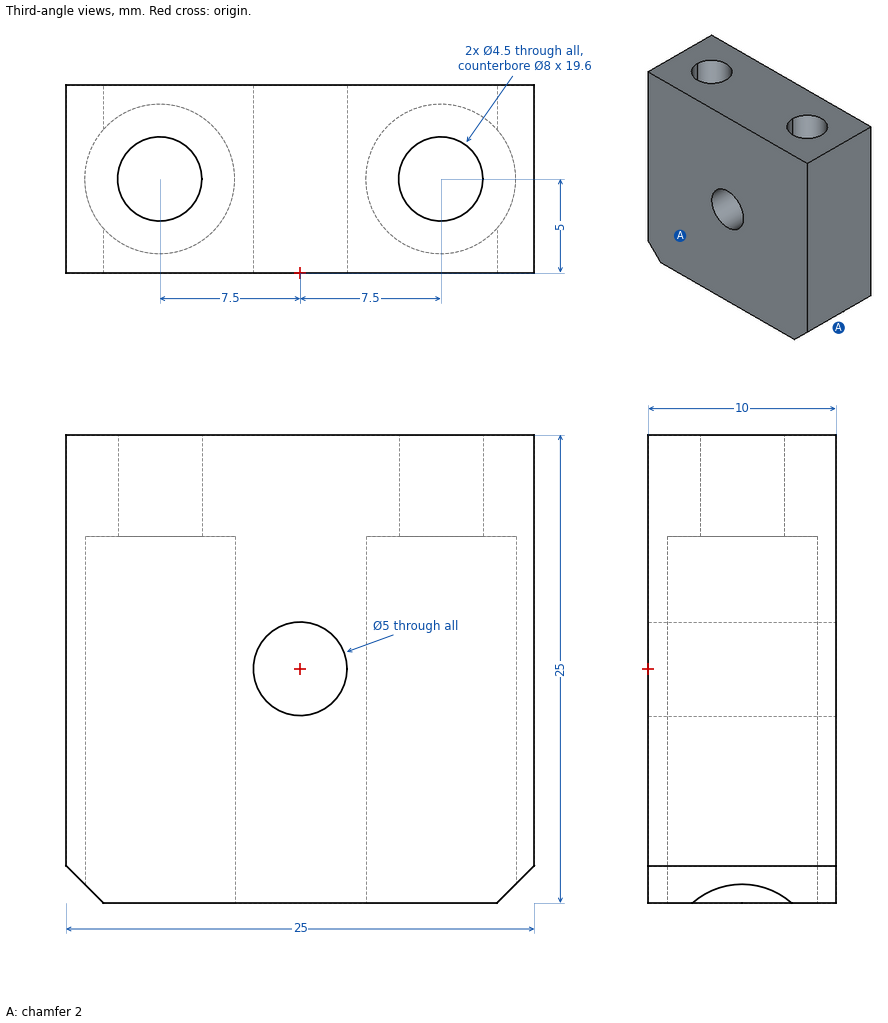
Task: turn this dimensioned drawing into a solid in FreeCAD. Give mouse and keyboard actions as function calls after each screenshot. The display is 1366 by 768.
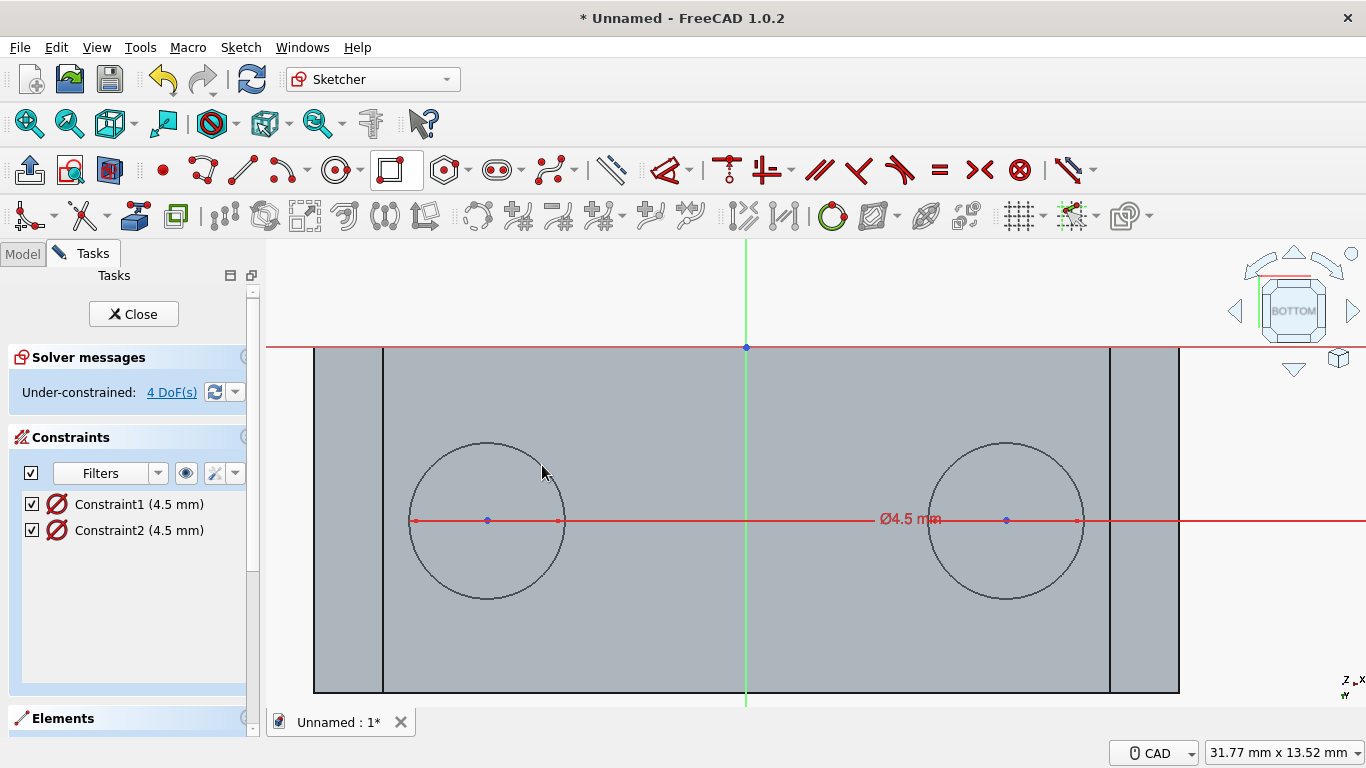
click(1006, 521)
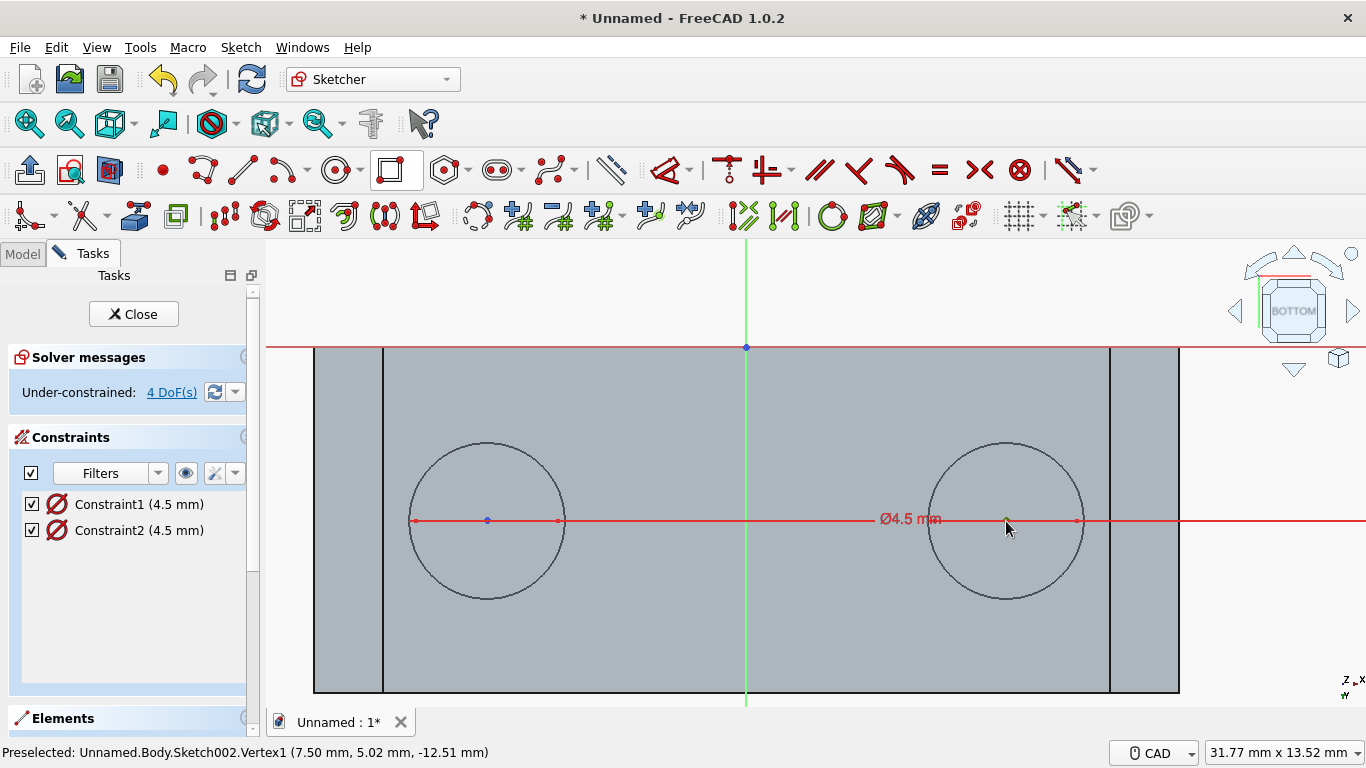
click(487, 521)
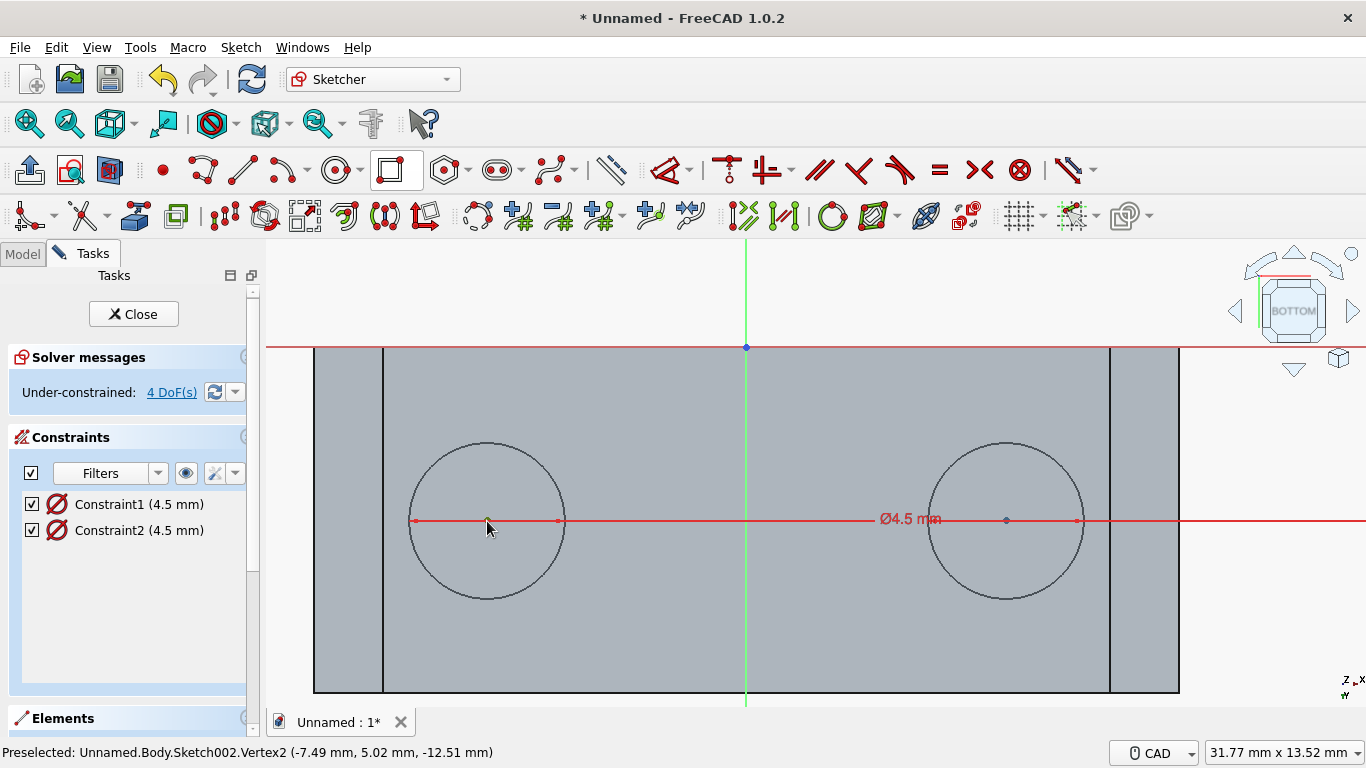
key(h)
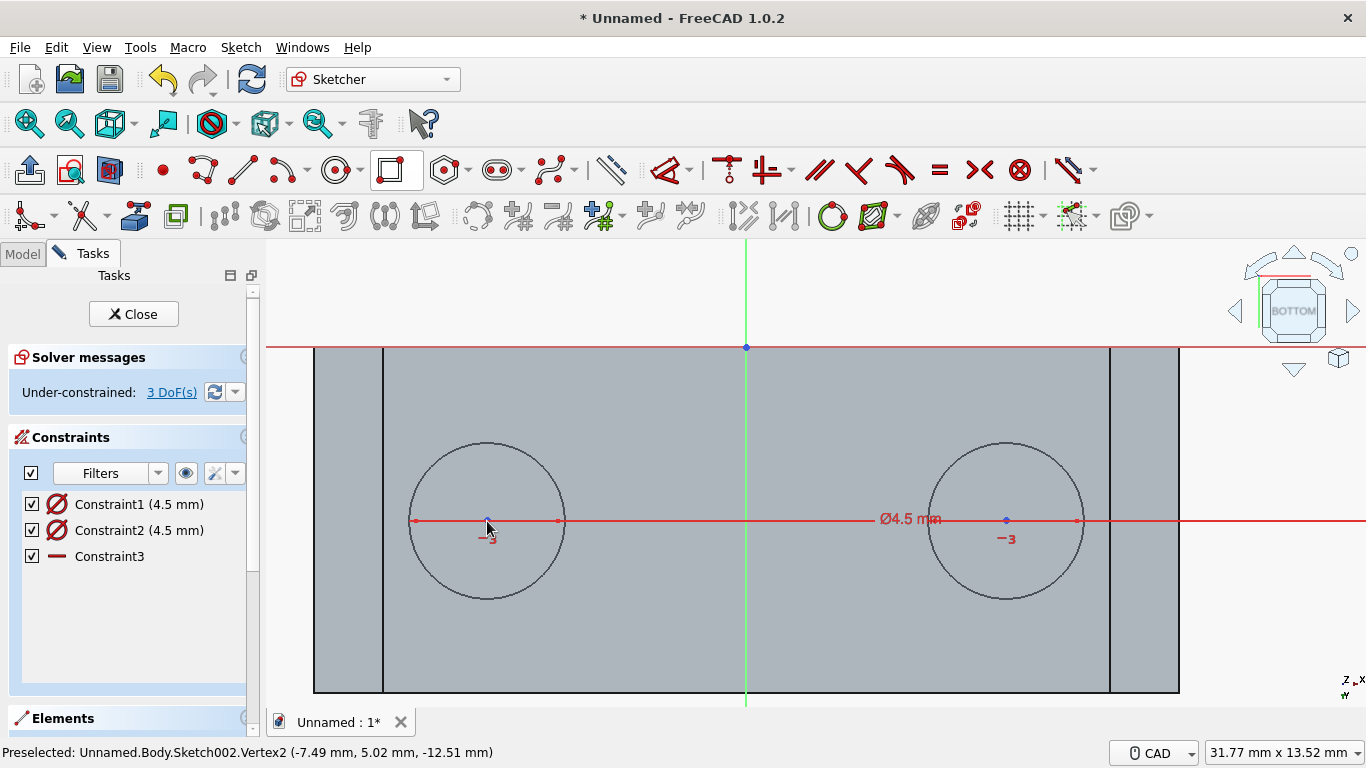
click(666, 170)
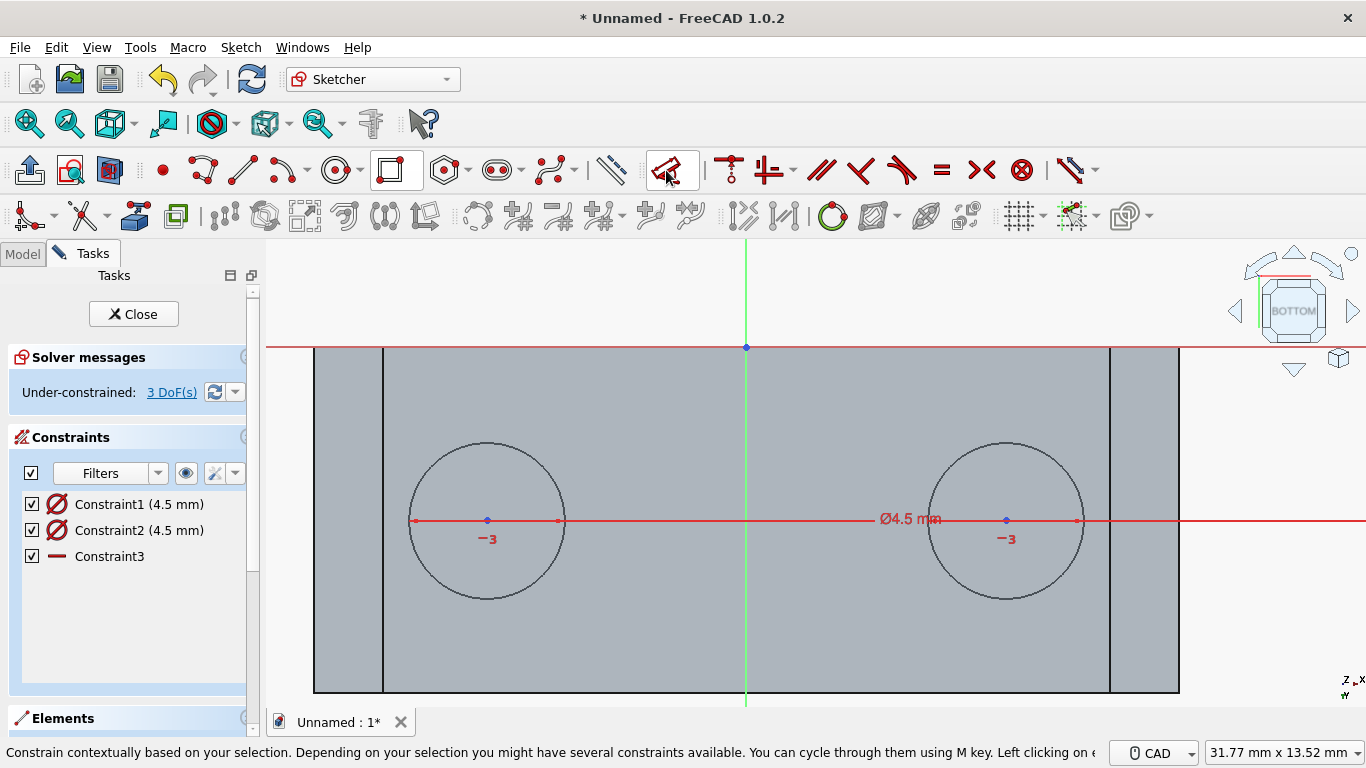
click(1006, 521)
click(1040, 434)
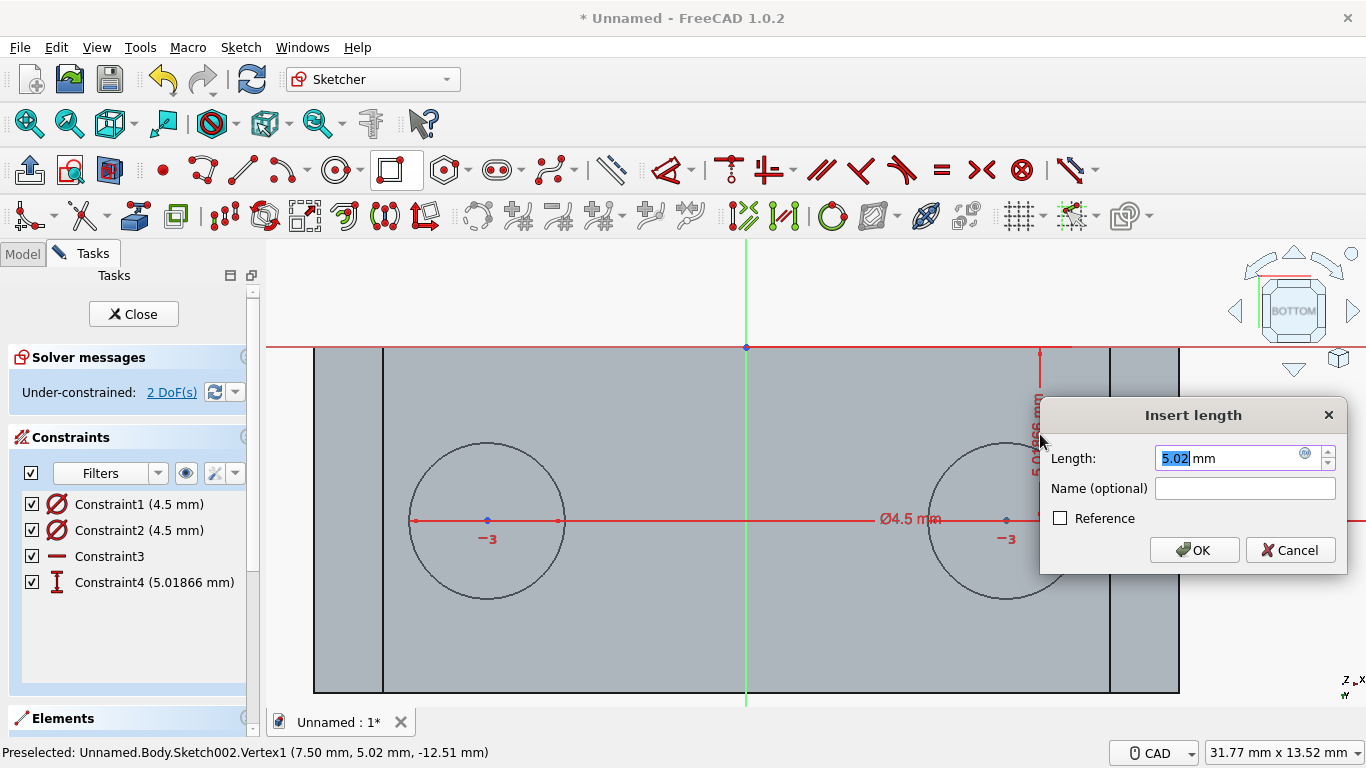
text(5)
key(Return)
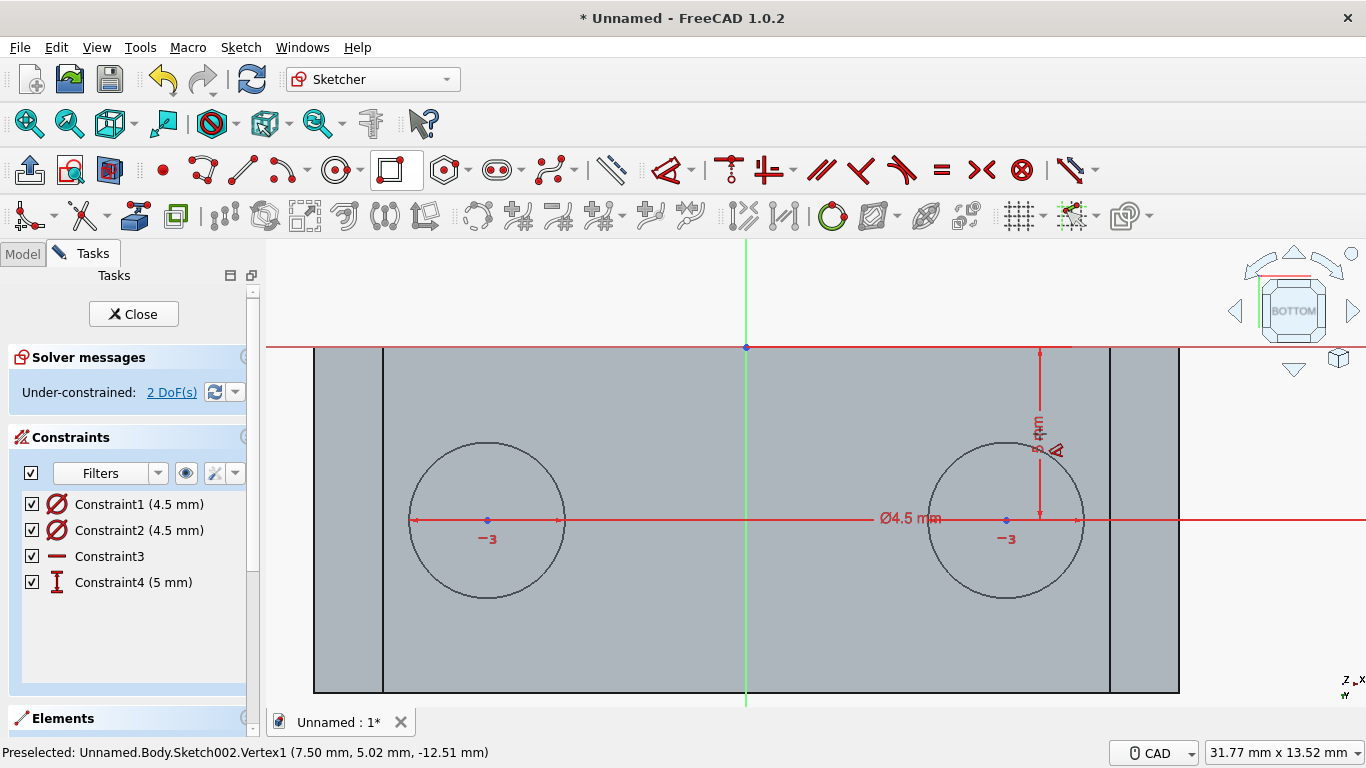
click(1006, 520)
click(876, 313)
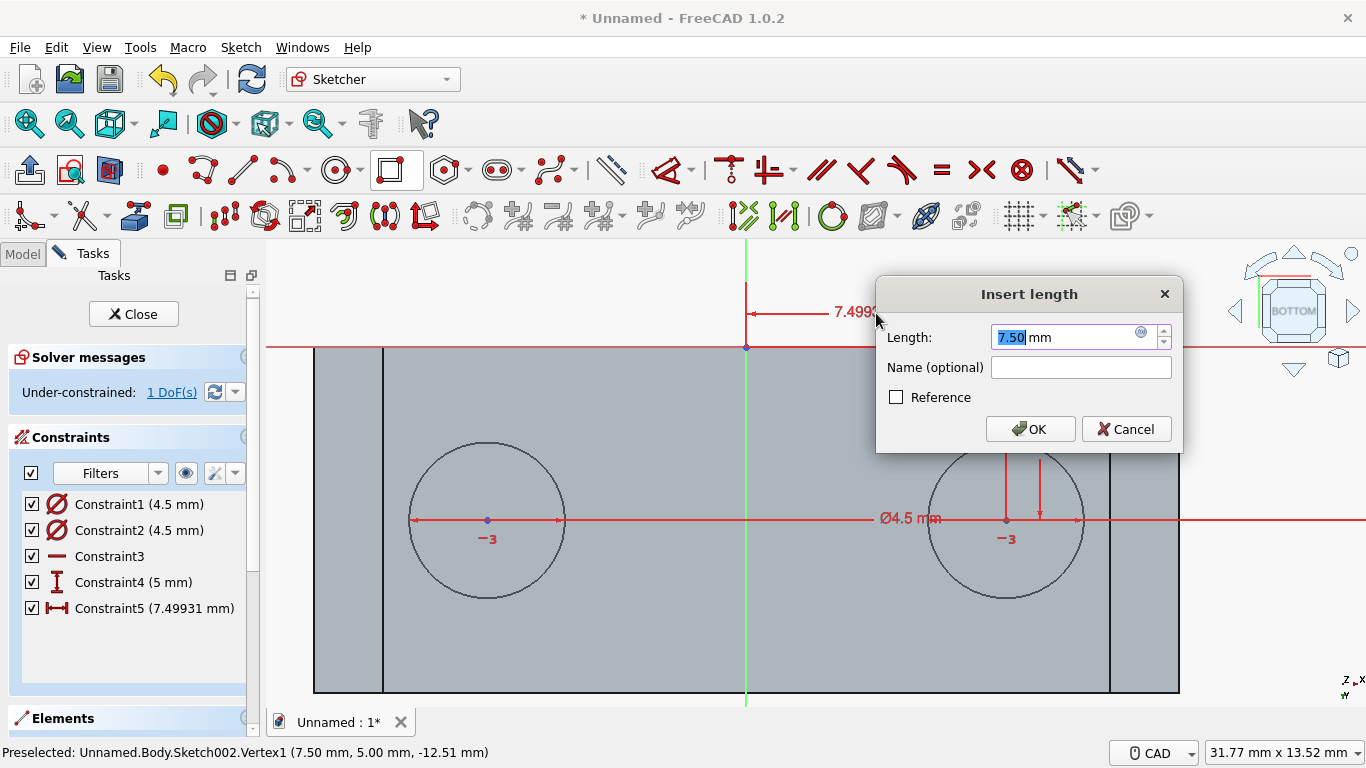
text(7.5)
key(Return)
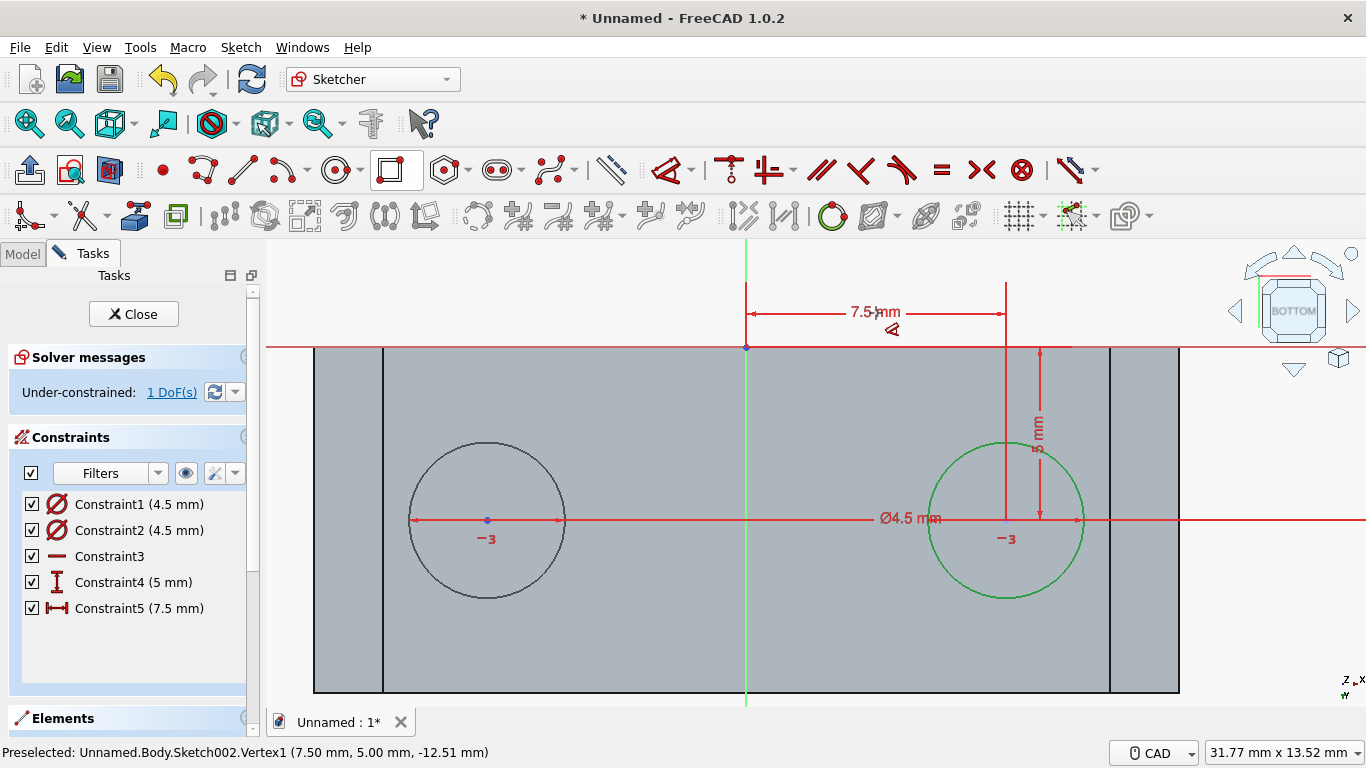
click(487, 520)
click(617, 313)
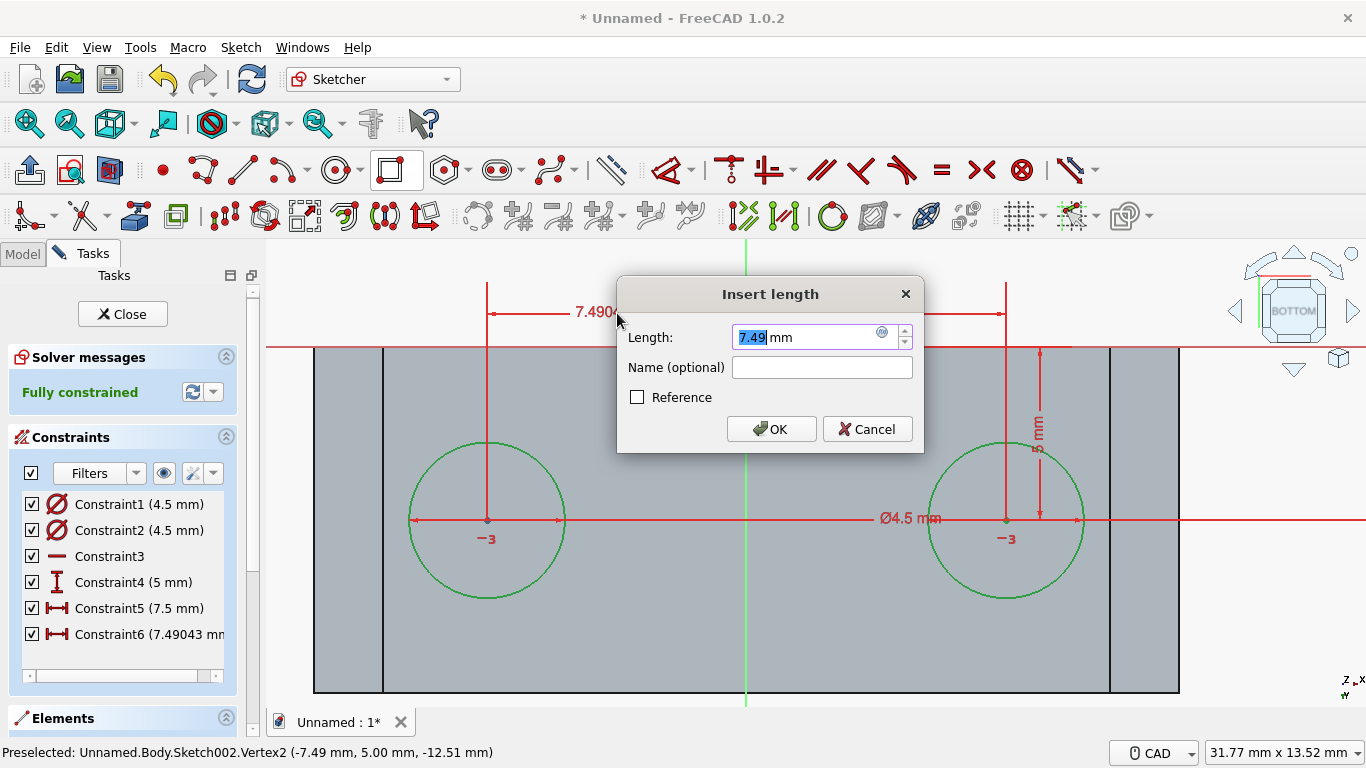
text(7.5)
key(Return)
key(Escape)